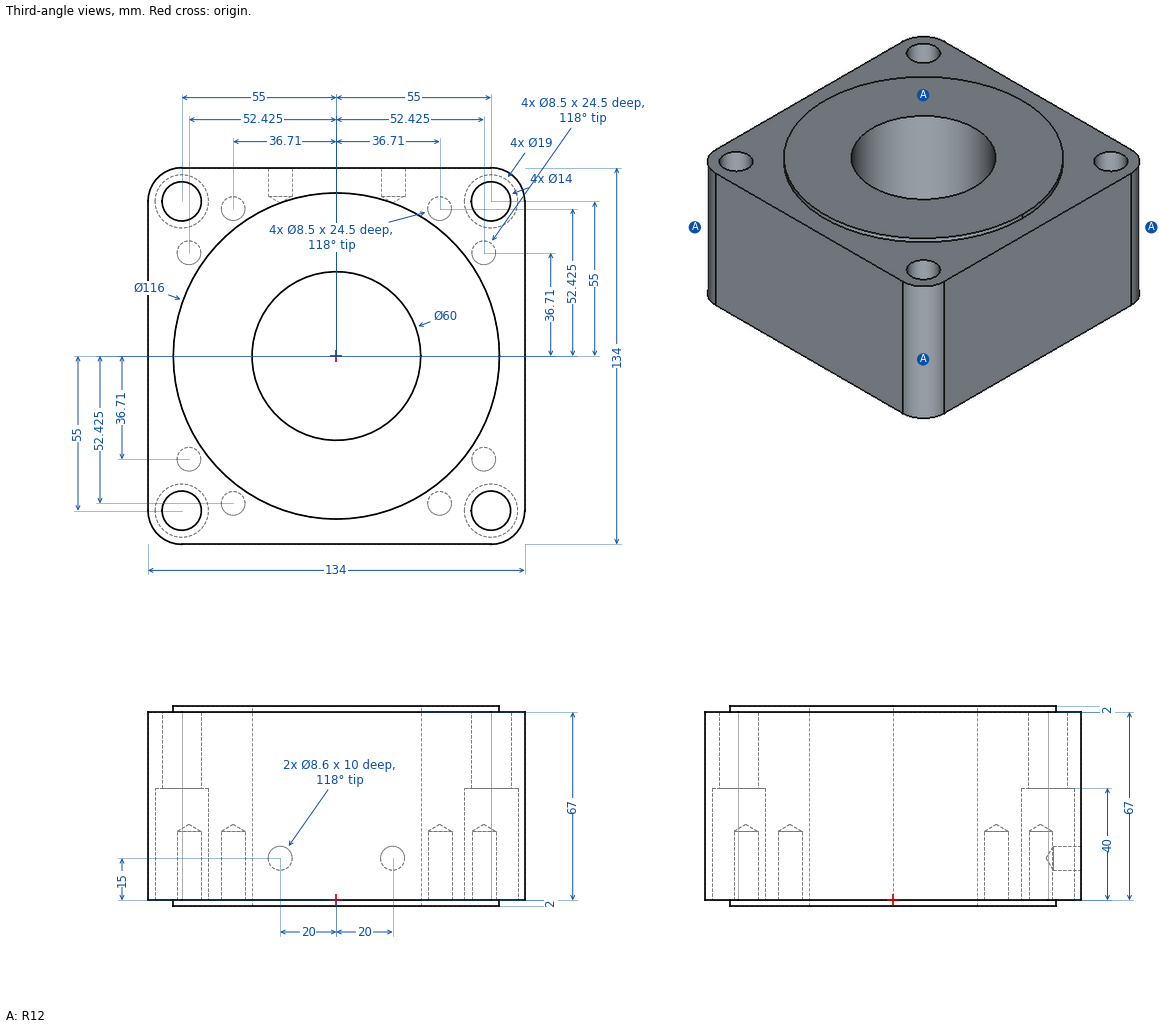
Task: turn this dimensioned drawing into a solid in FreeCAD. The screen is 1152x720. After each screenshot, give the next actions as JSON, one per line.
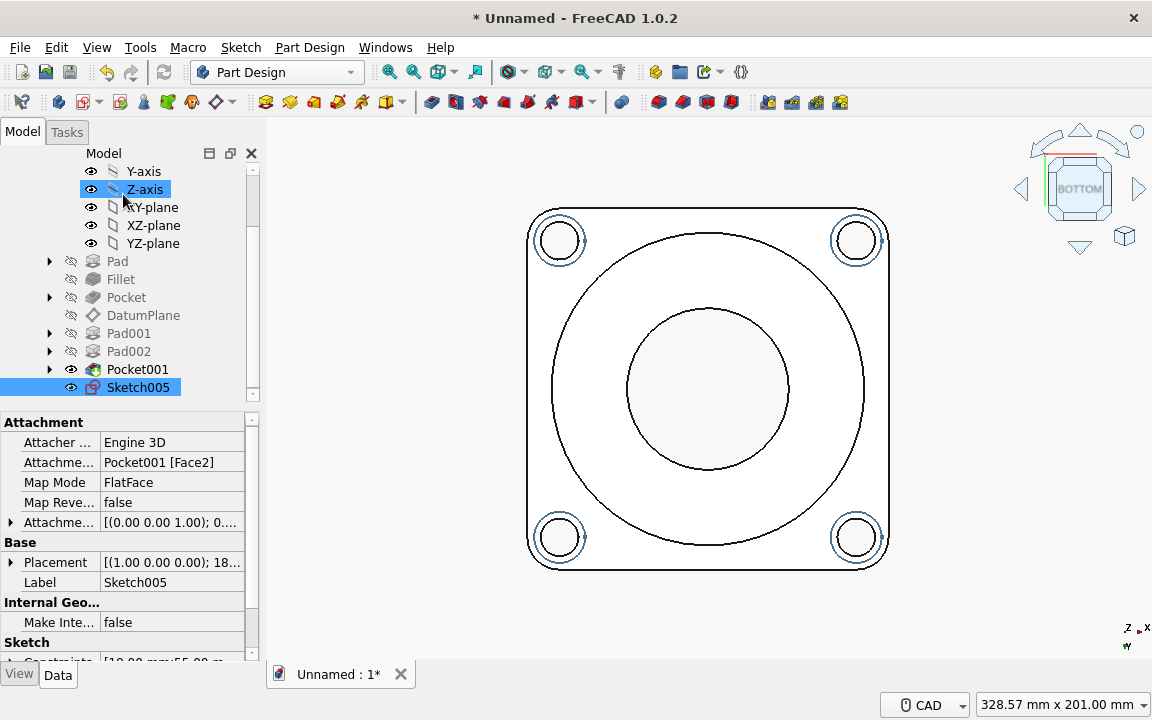
{"action": "left_click", "coordinate": [432, 102]}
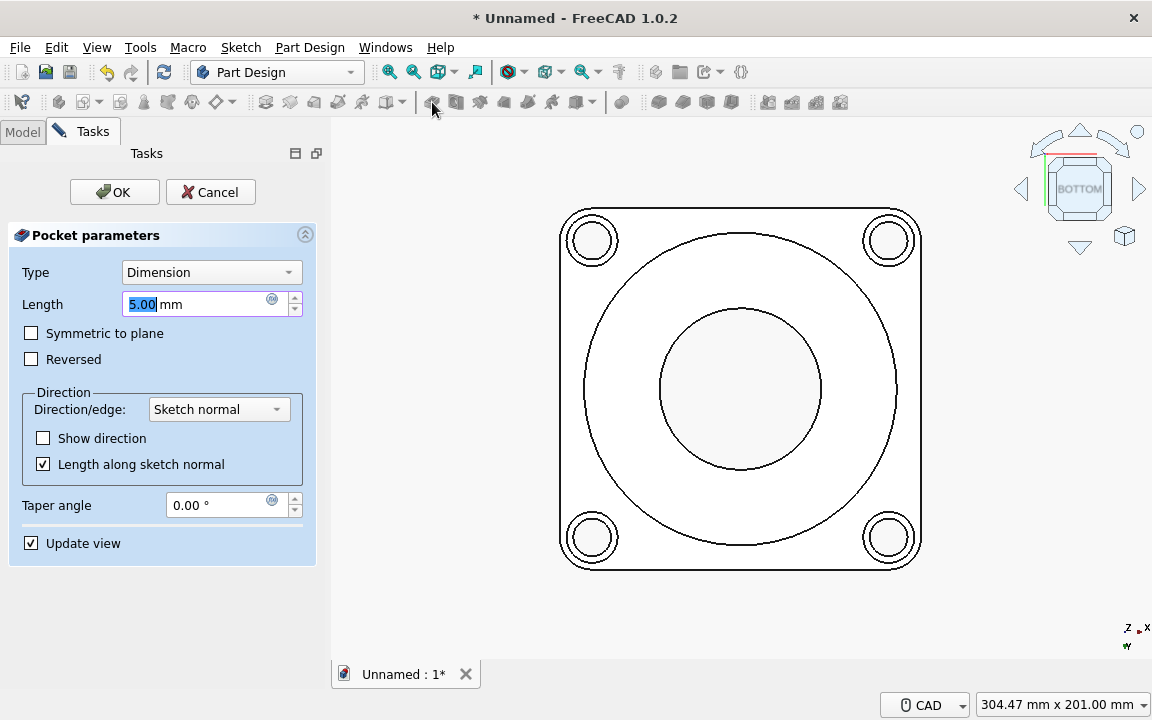
{"action": "type", "text": "40"}
{"action": "key", "text": "Tab"}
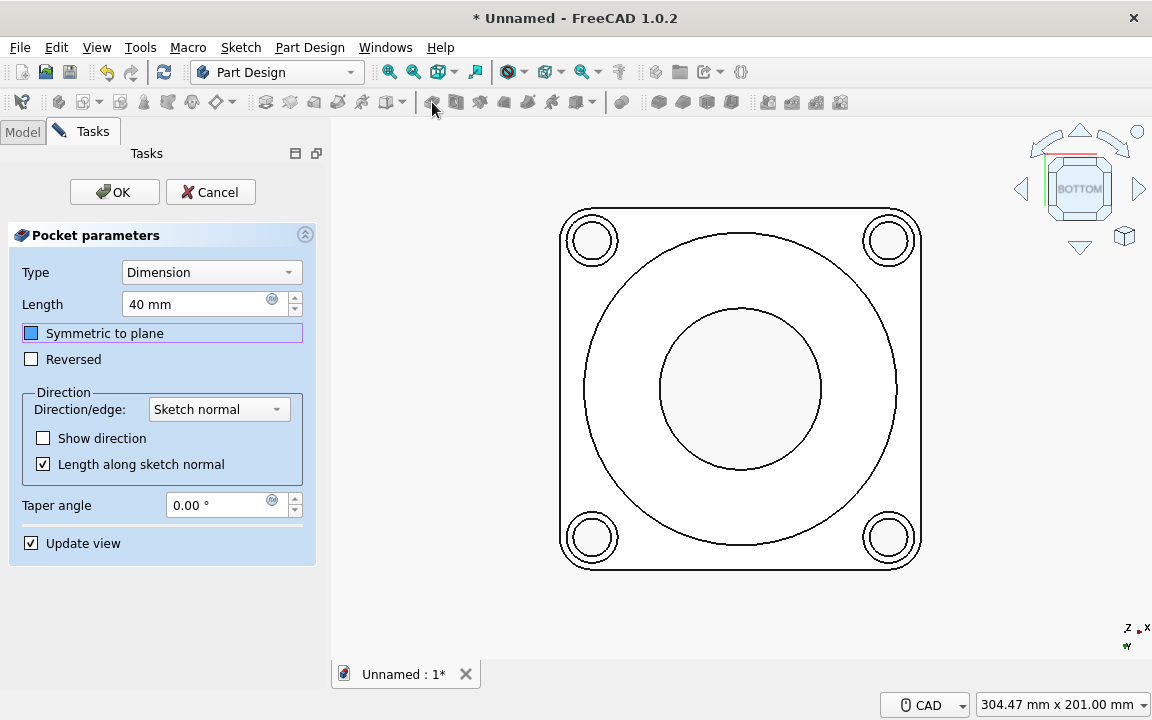
{"action": "left_click", "coordinate": [115, 192]}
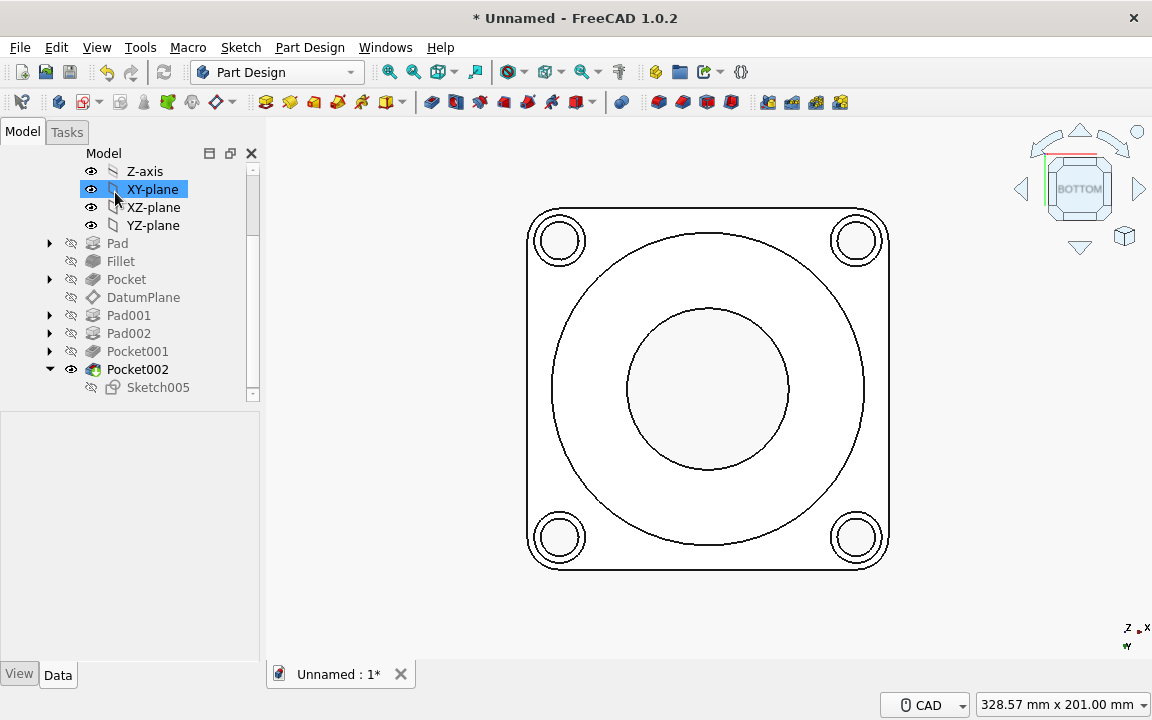
{"action": "left_click", "coordinate": [863, 285]}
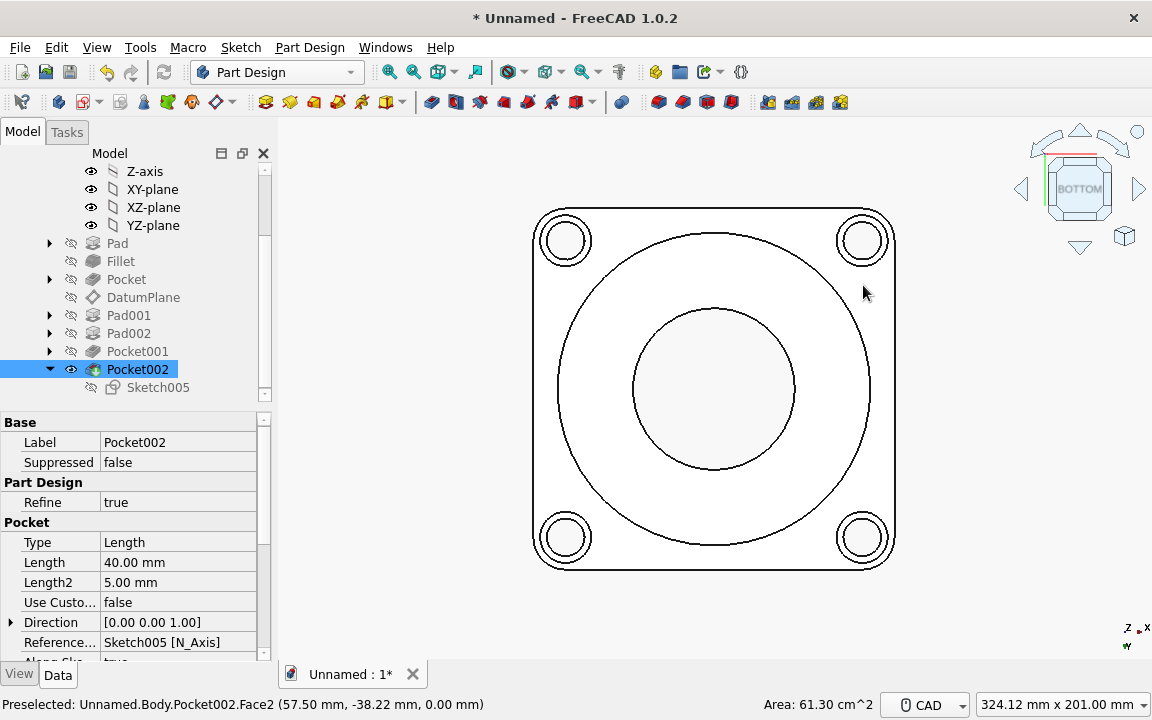
{"action": "left_click", "coordinate": [84, 102]}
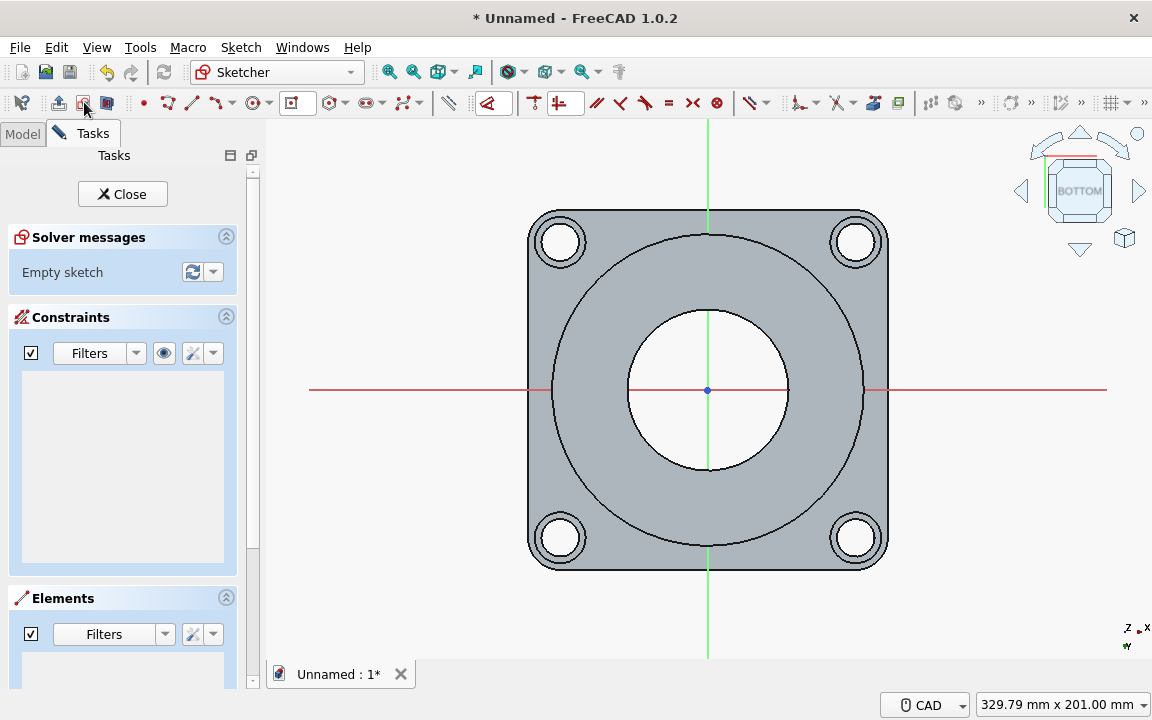
{"action": "left_click", "coordinate": [254, 104]}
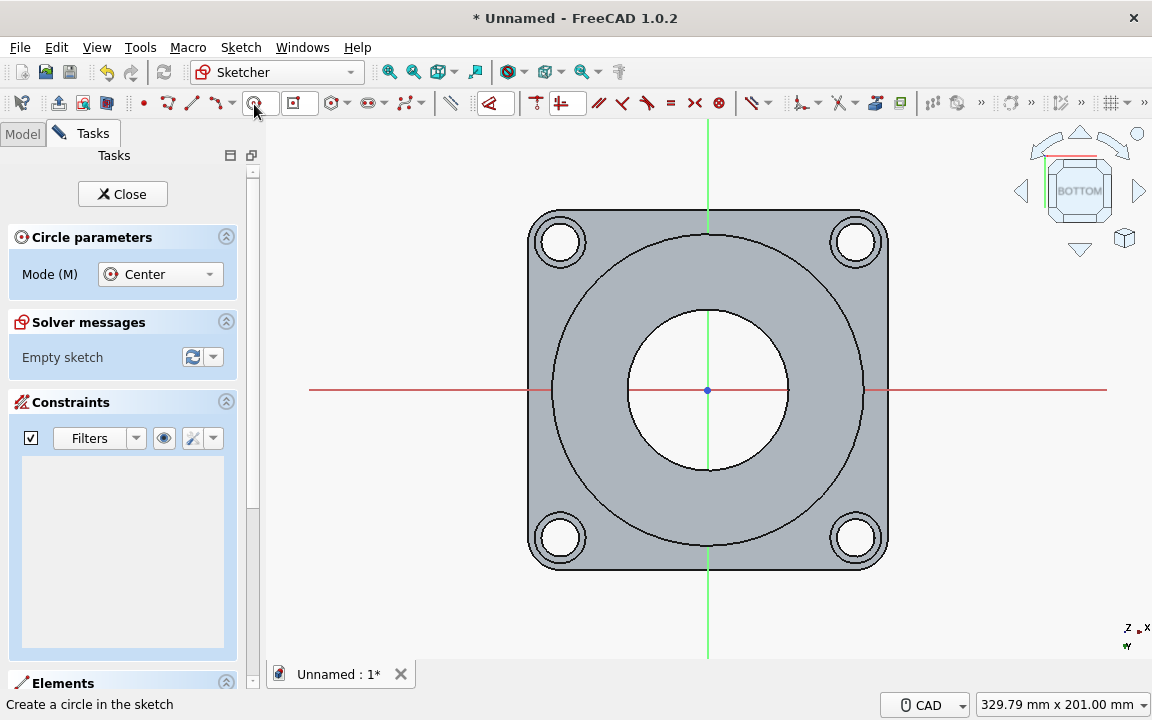
{"action": "scroll", "coordinate": [807, 531], "scroll_direction": "up", "scroll_amount": 4}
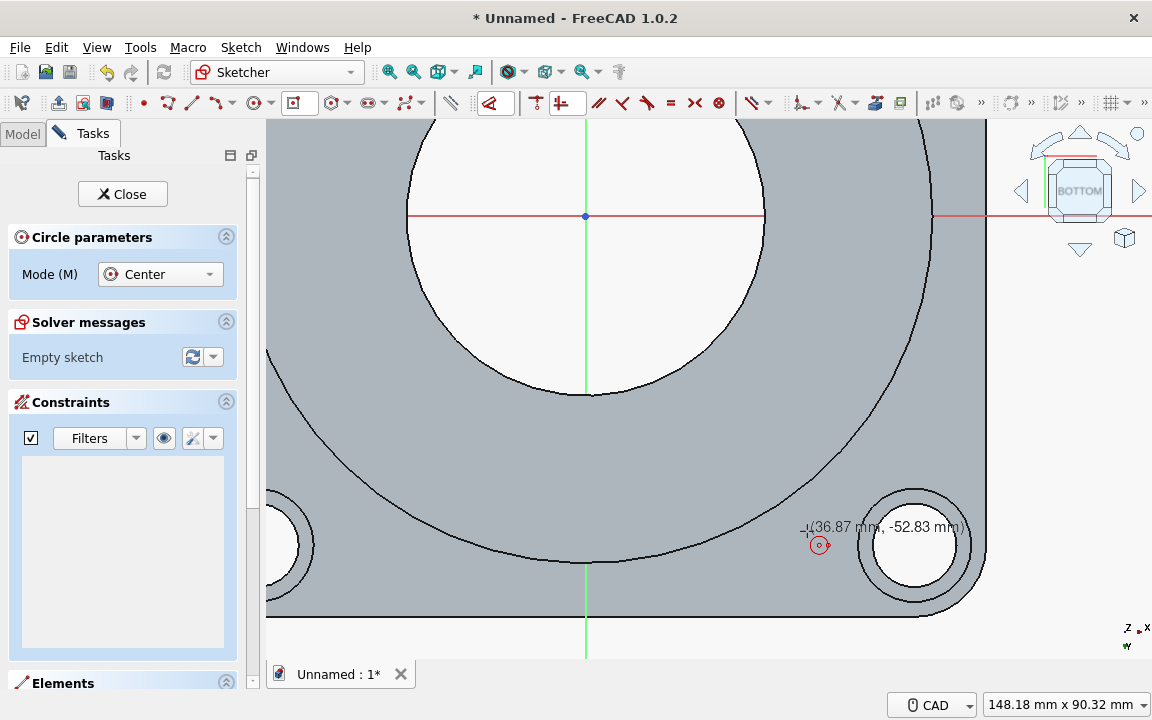
{"action": "left_click", "coordinate": [805, 530]}
{"action": "left_click", "coordinate": [823, 512]}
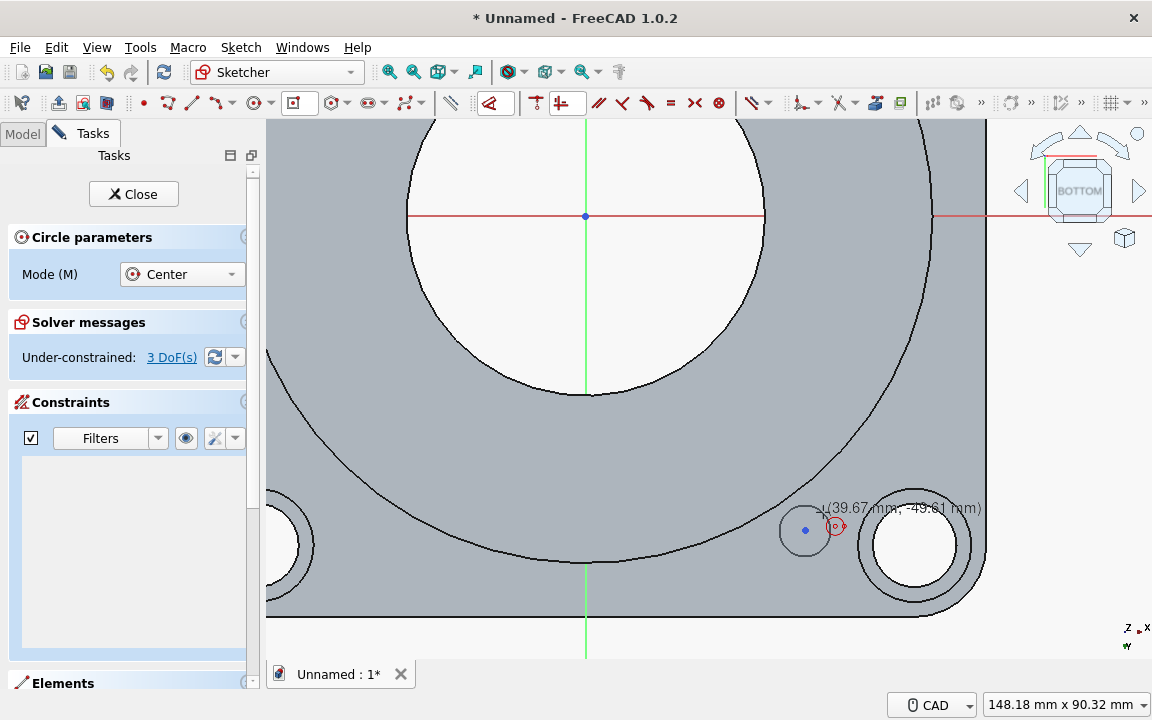
{"action": "left_click", "coordinate": [366, 530]}
{"action": "left_click", "coordinate": [384, 512]}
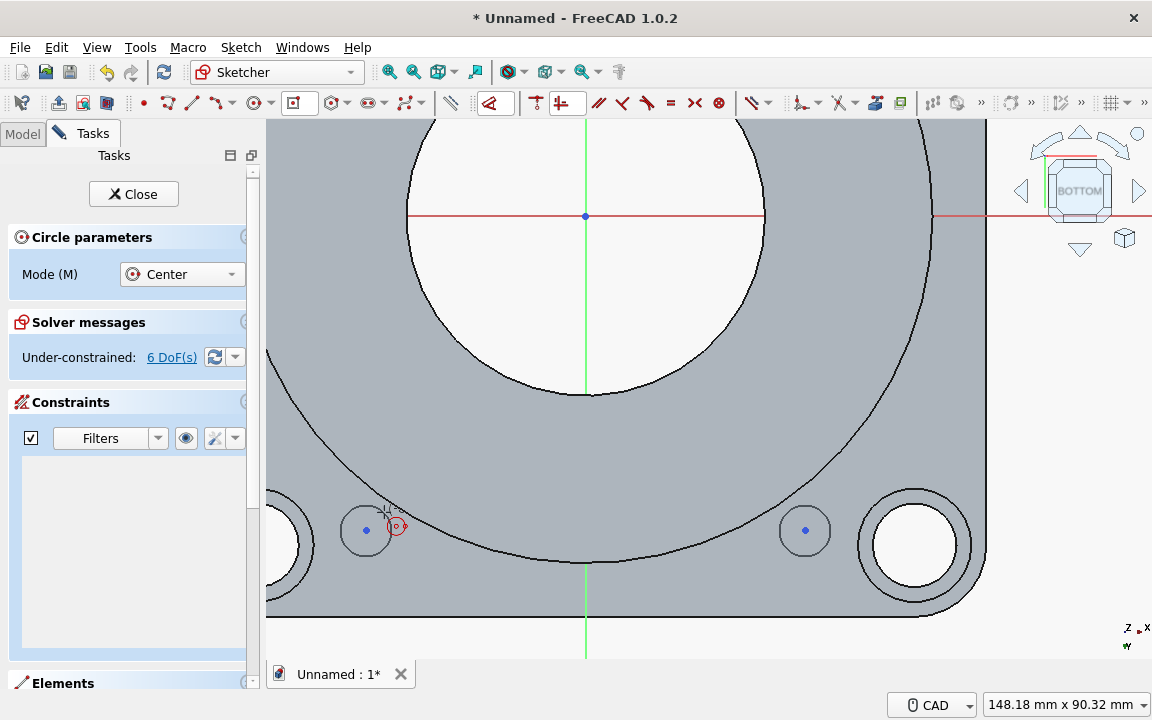
{"action": "scroll", "coordinate": [707, 599], "scroll_direction": "down", "scroll_amount": 3}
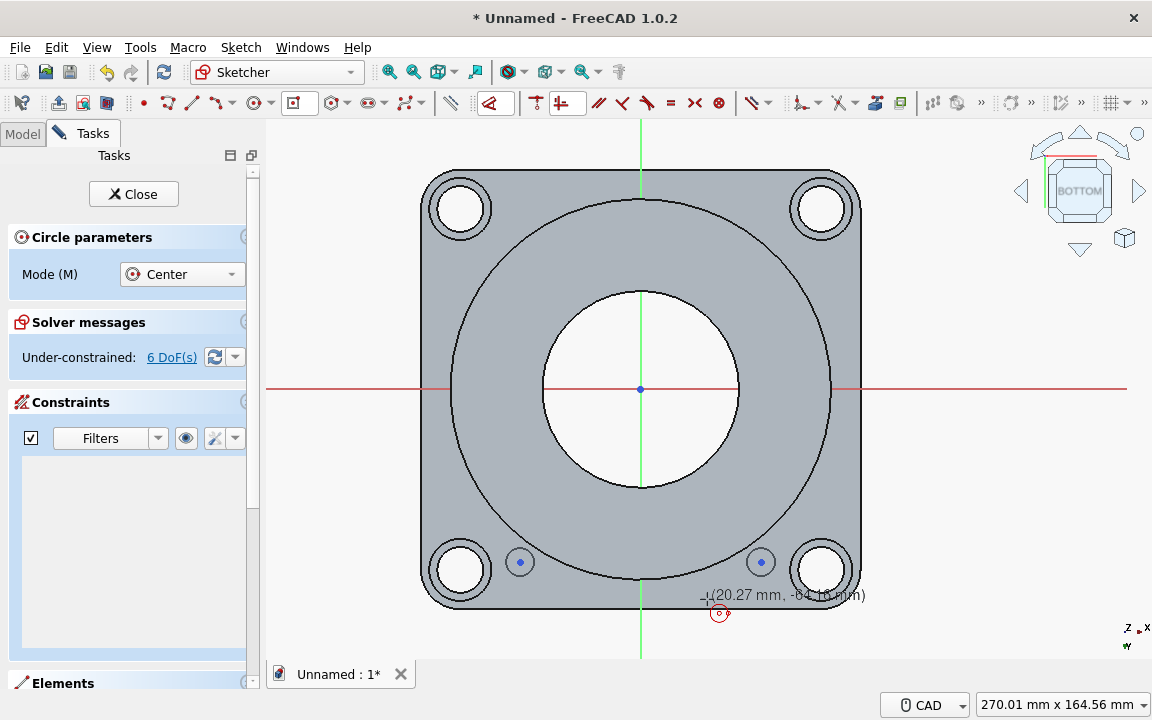
{"action": "scroll", "coordinate": [520, 217], "scroll_direction": "up", "scroll_amount": 3}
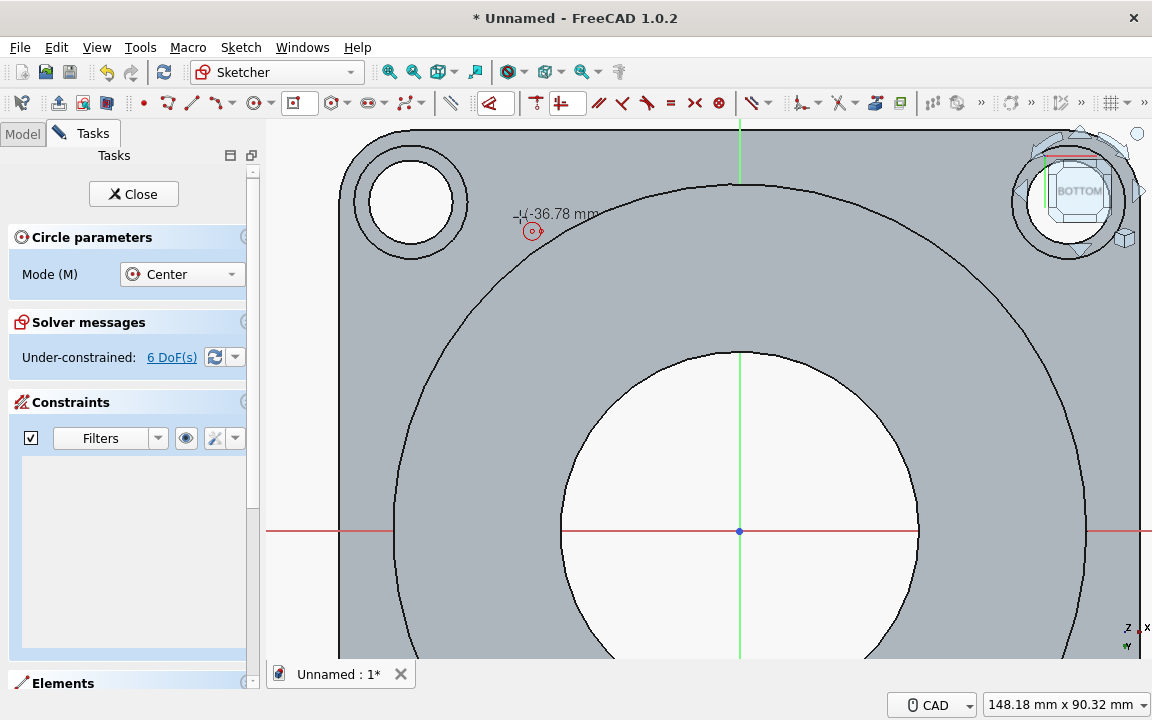
{"action": "left_click", "coordinate": [520, 218]}
{"action": "left_click", "coordinate": [538, 200]}